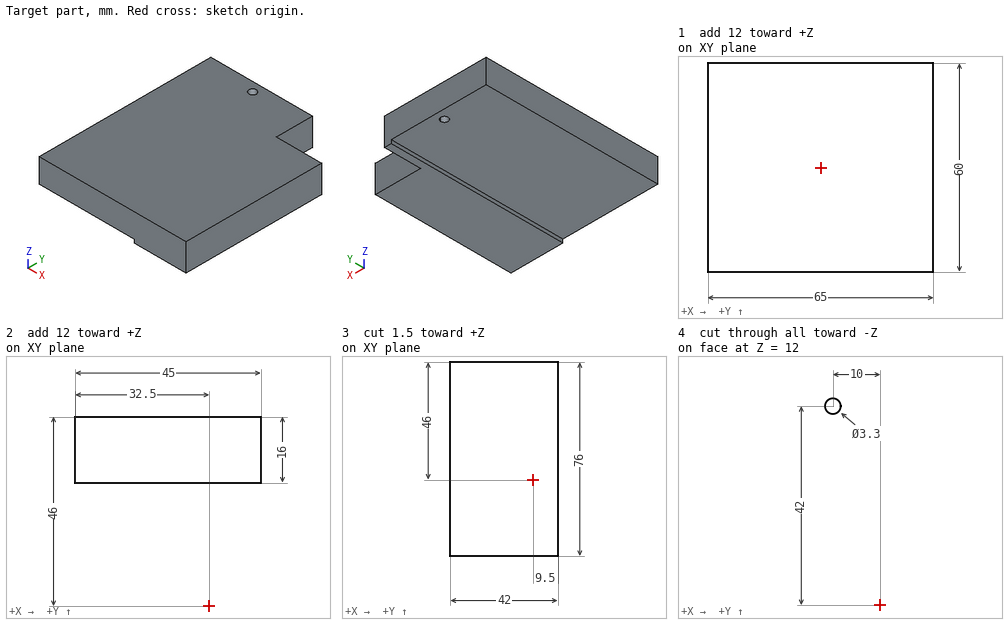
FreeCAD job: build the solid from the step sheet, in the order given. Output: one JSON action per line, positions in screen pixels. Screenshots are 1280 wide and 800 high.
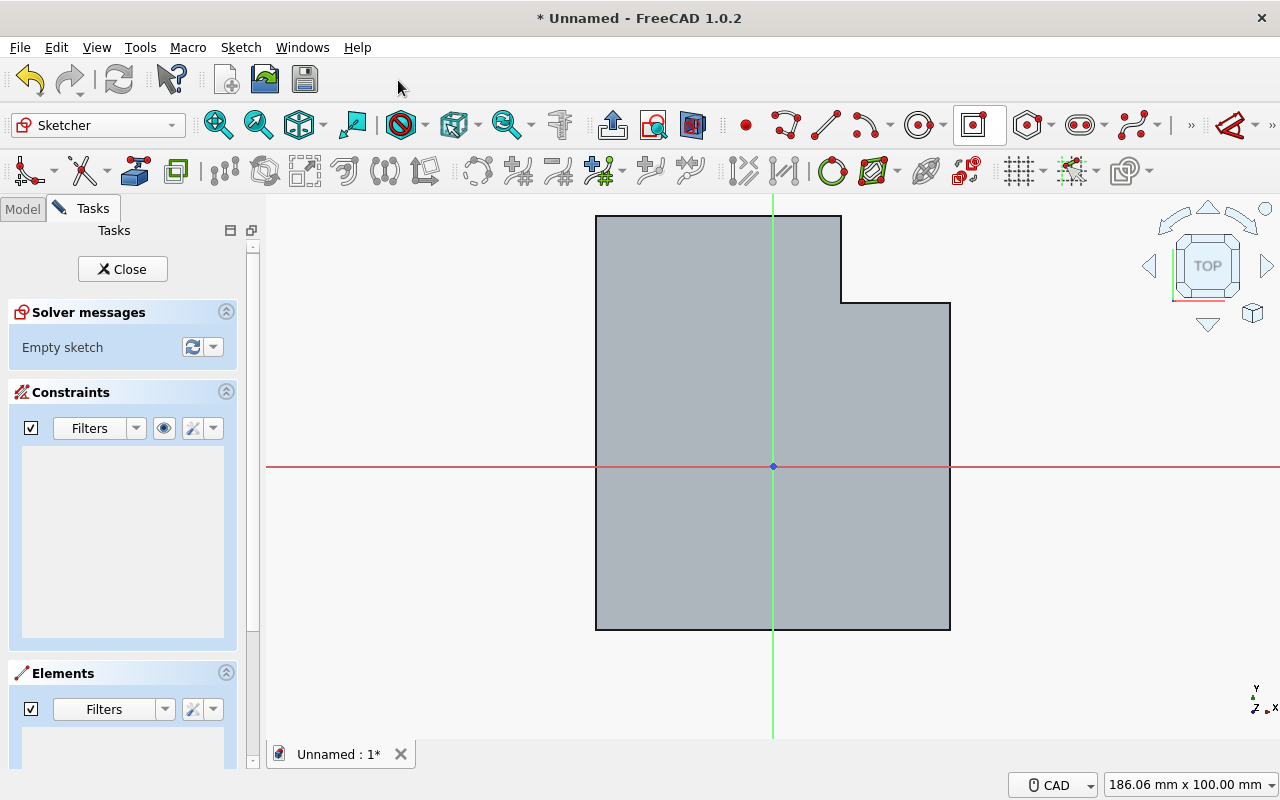
{"action": "scroll", "coordinate": [719, 226], "scroll_direction": "up", "scroll_amount": 15}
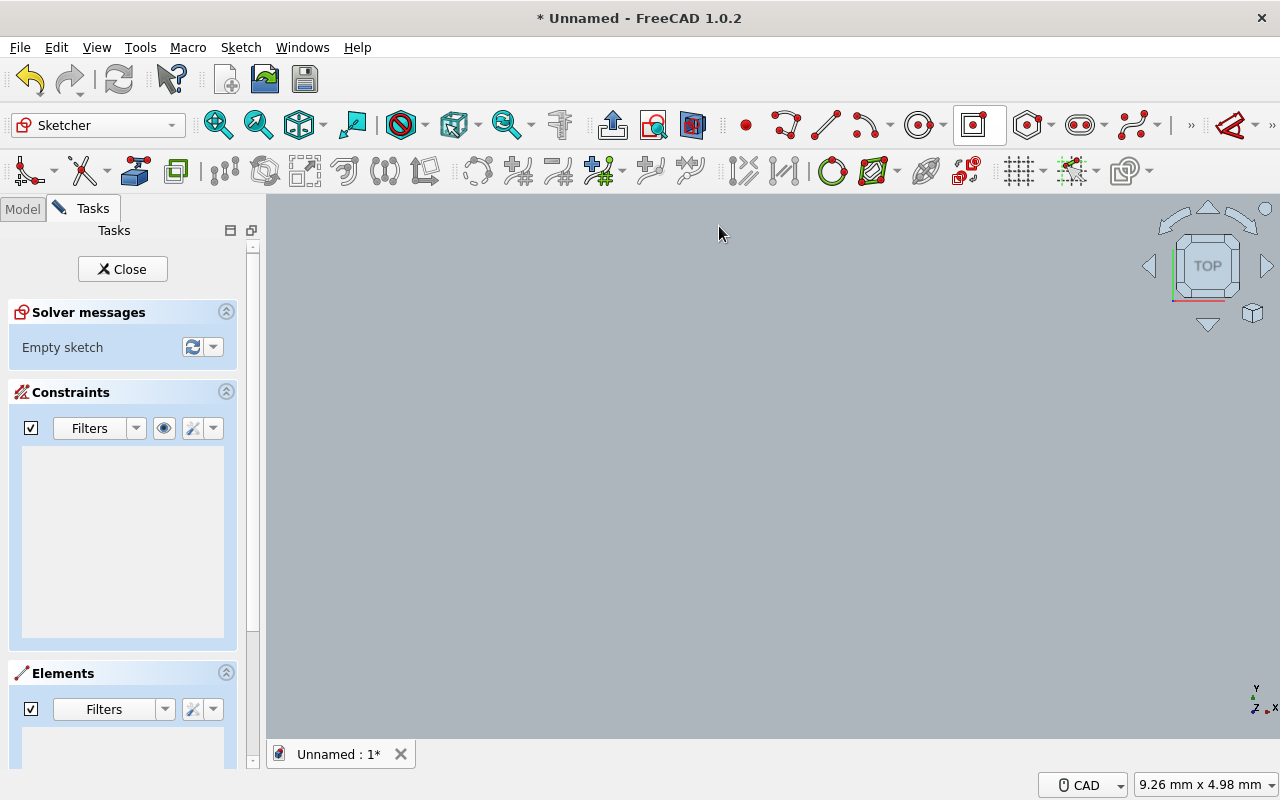
{"action": "left_click", "coordinate": [920, 126]}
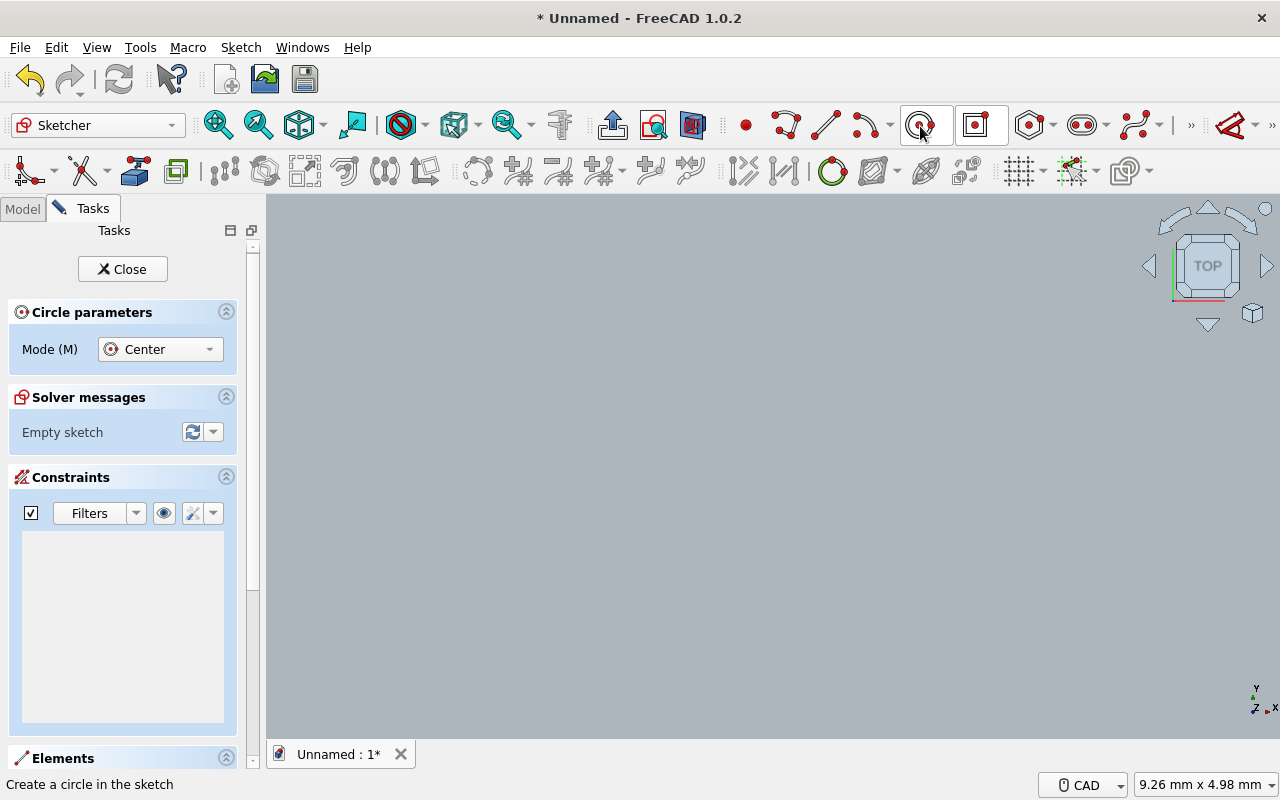
{"action": "left_click", "coordinate": [700, 458]}
{"action": "mouse_move", "coordinate": [828, 330]}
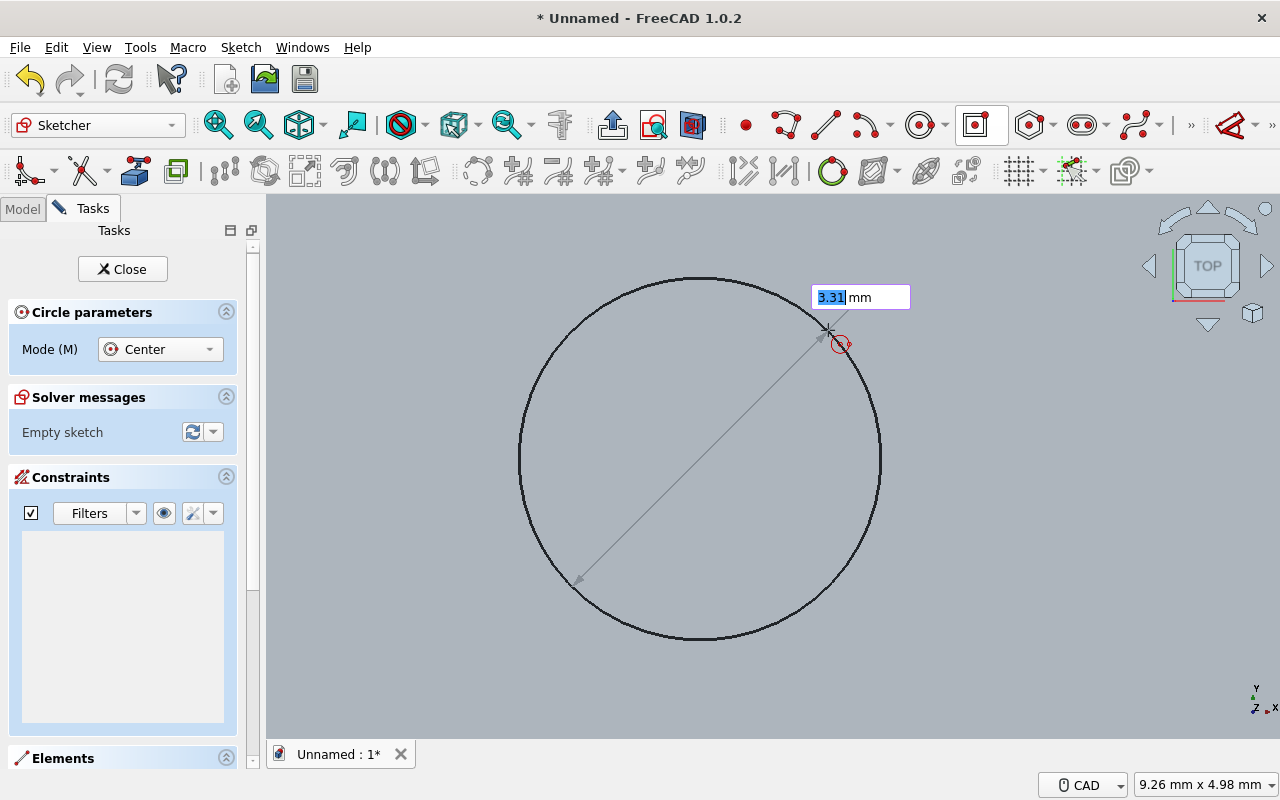
{"action": "type", "text": "3.3"}
{"action": "key", "text": "Return"}
{"action": "key", "text": "Escape"}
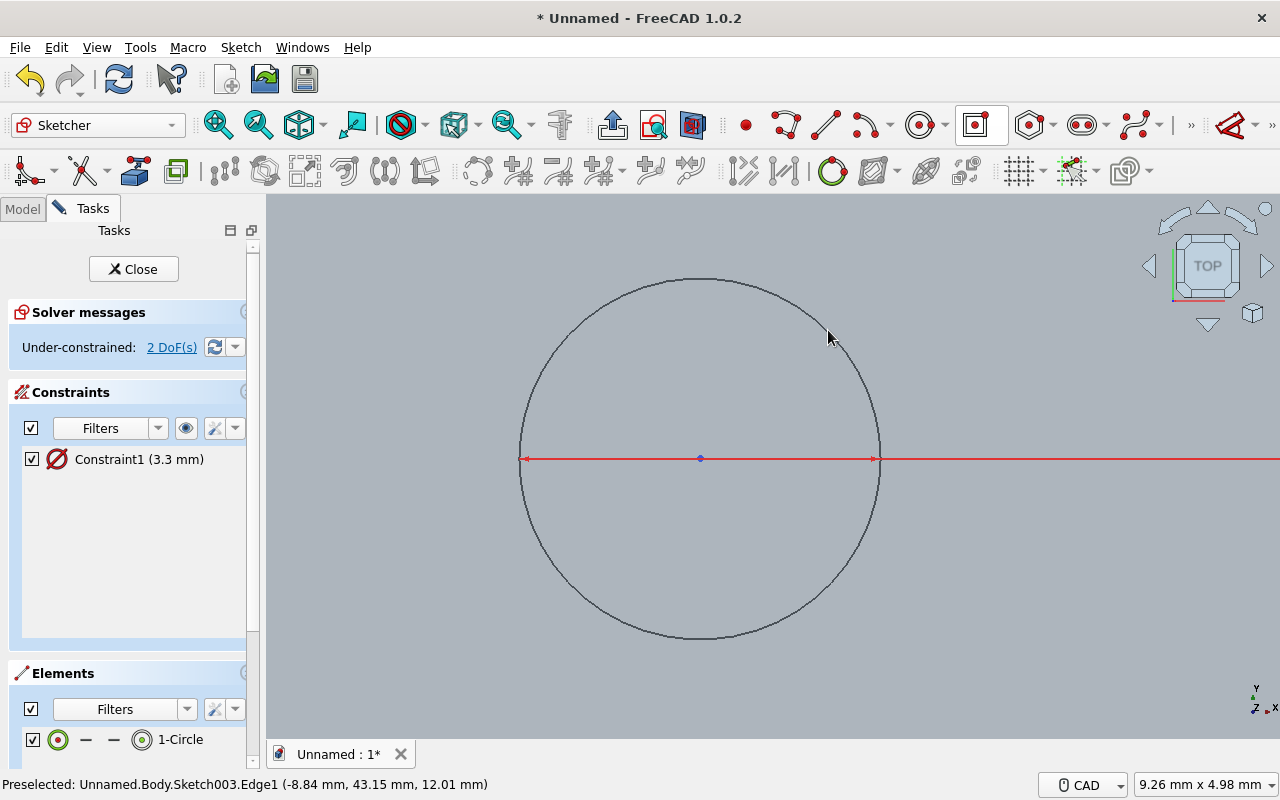
{"action": "left_click", "coordinate": [1230, 126]}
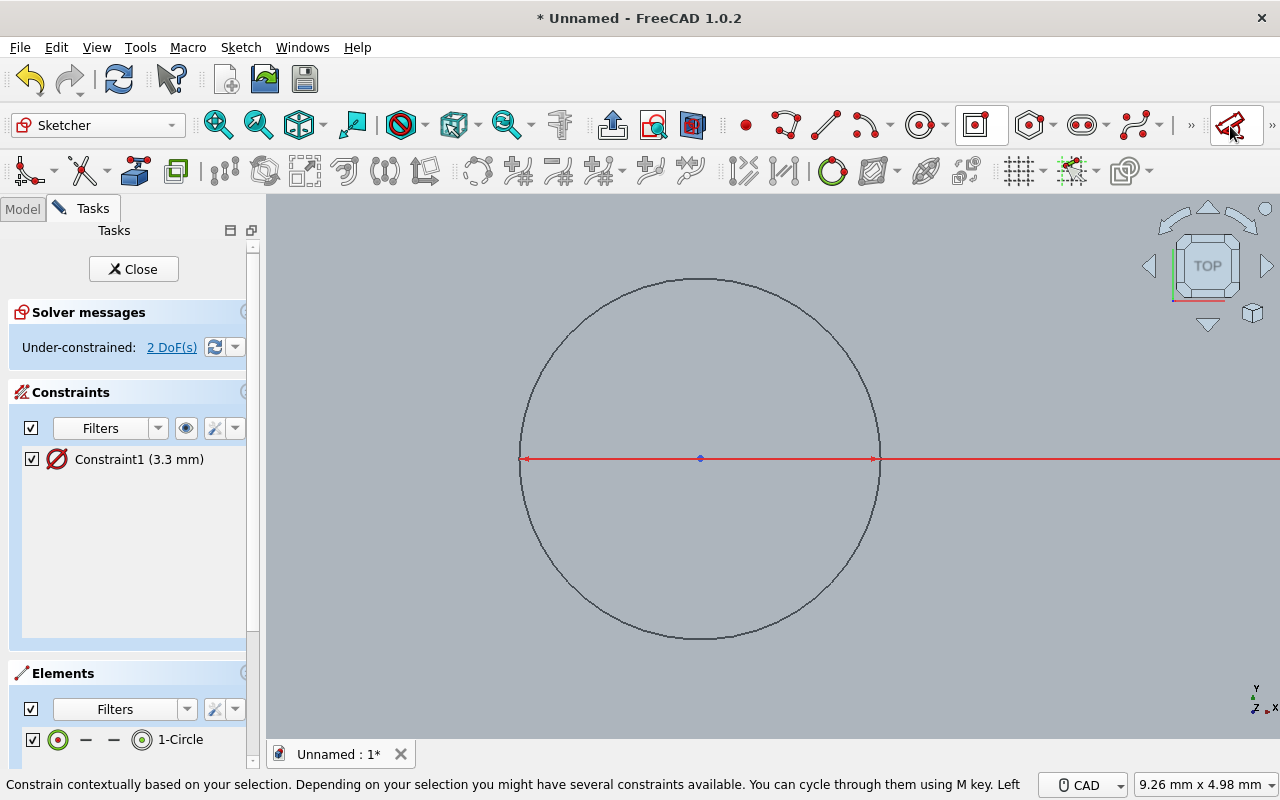
{"action": "left_click", "coordinate": [700, 459]}
{"action": "left_click", "coordinate": [907, 425]}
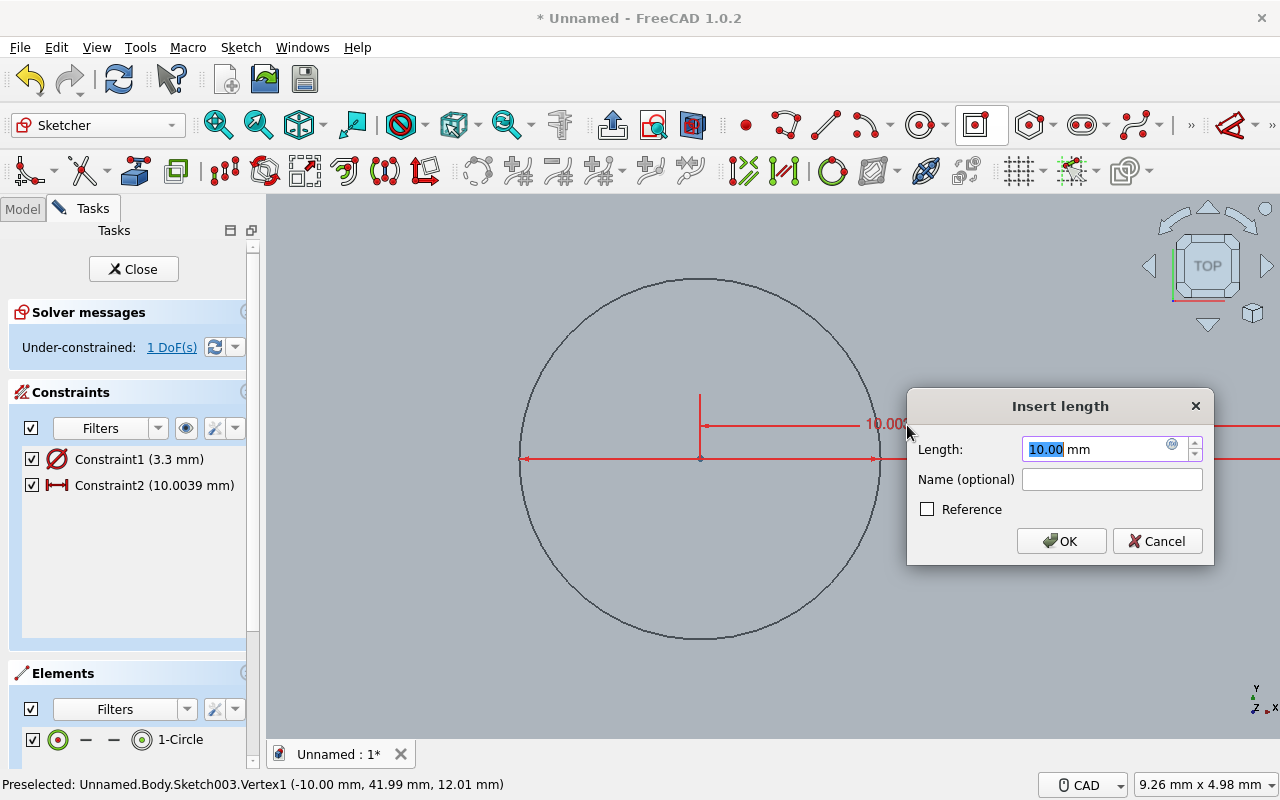
{"action": "type", "text": "10"}
{"action": "key", "text": "Return"}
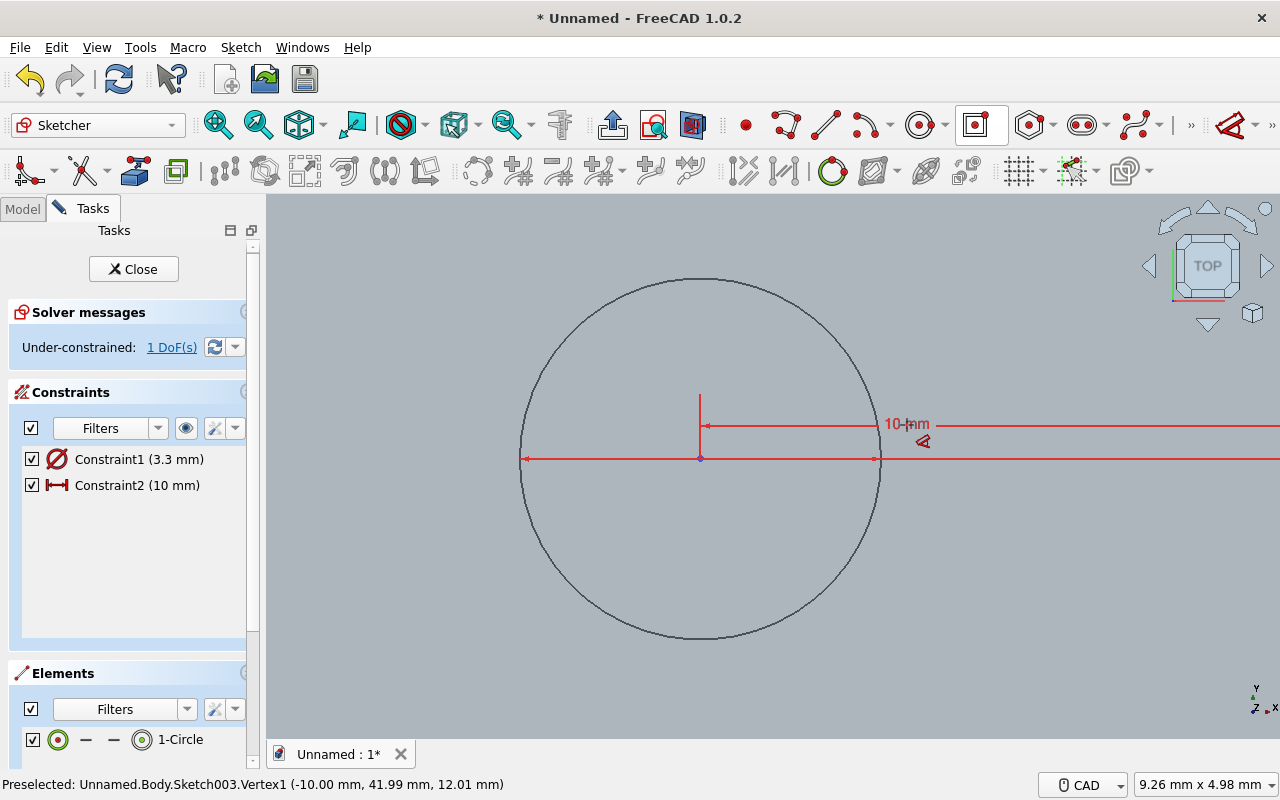
{"action": "left_click", "coordinate": [700, 459]}
{"action": "left_click", "coordinate": [666, 585]}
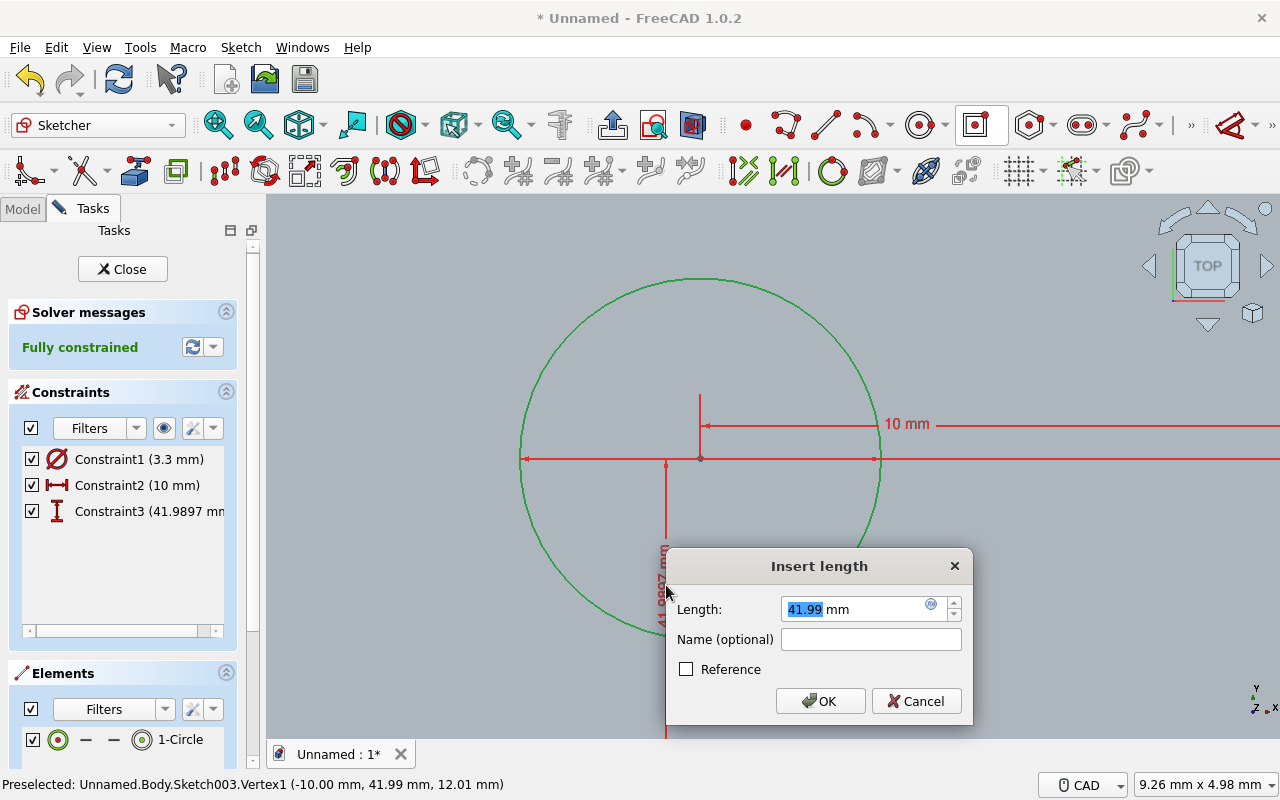
{"action": "type", "text": "42"}
{"action": "key", "text": "Return"}
{"action": "key", "text": "Escape"}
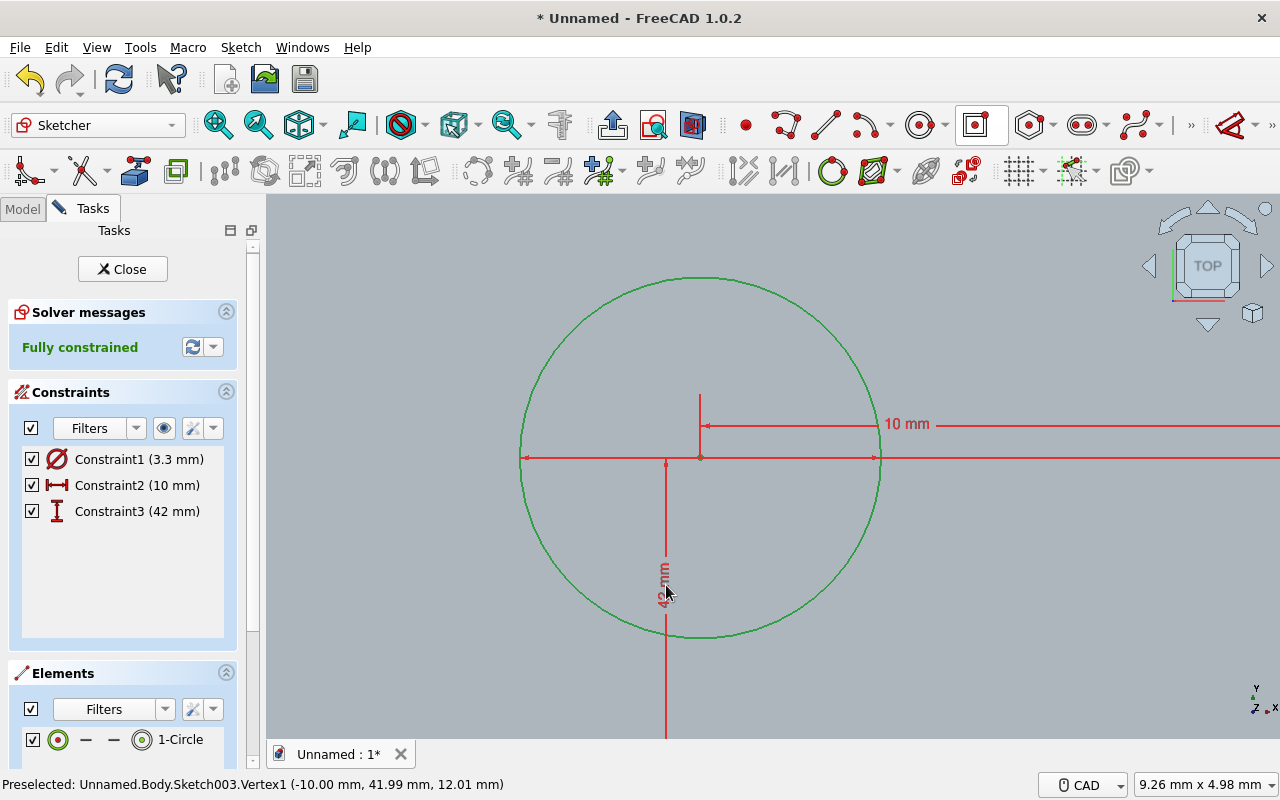
{"action": "left_click", "coordinate": [123, 269]}